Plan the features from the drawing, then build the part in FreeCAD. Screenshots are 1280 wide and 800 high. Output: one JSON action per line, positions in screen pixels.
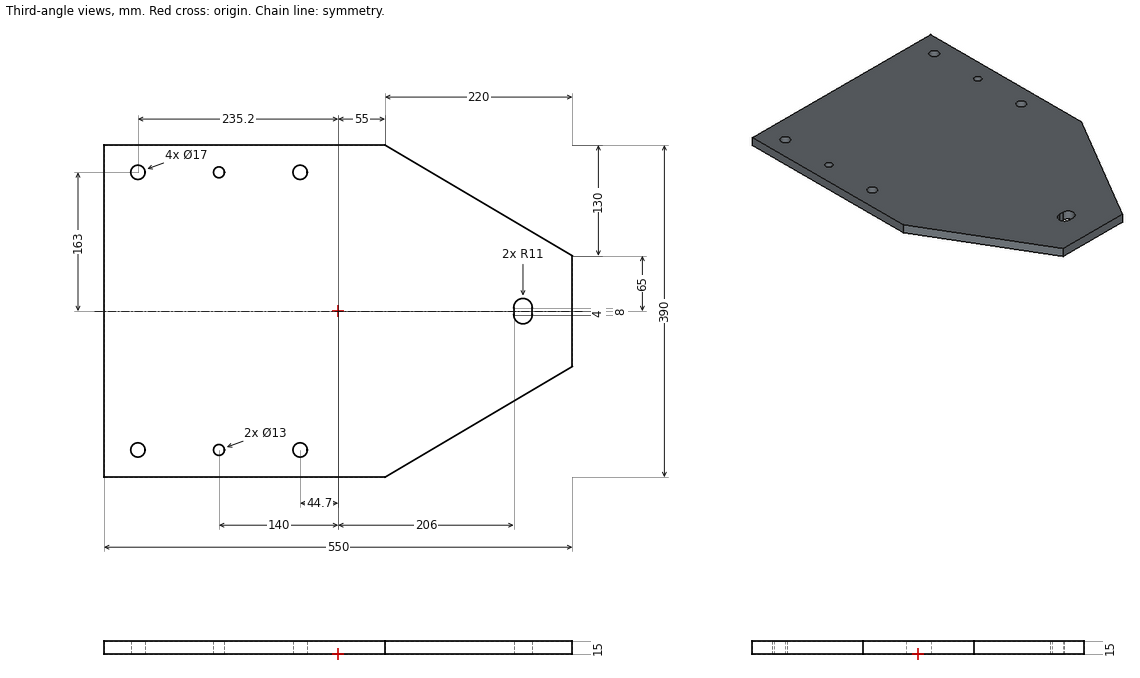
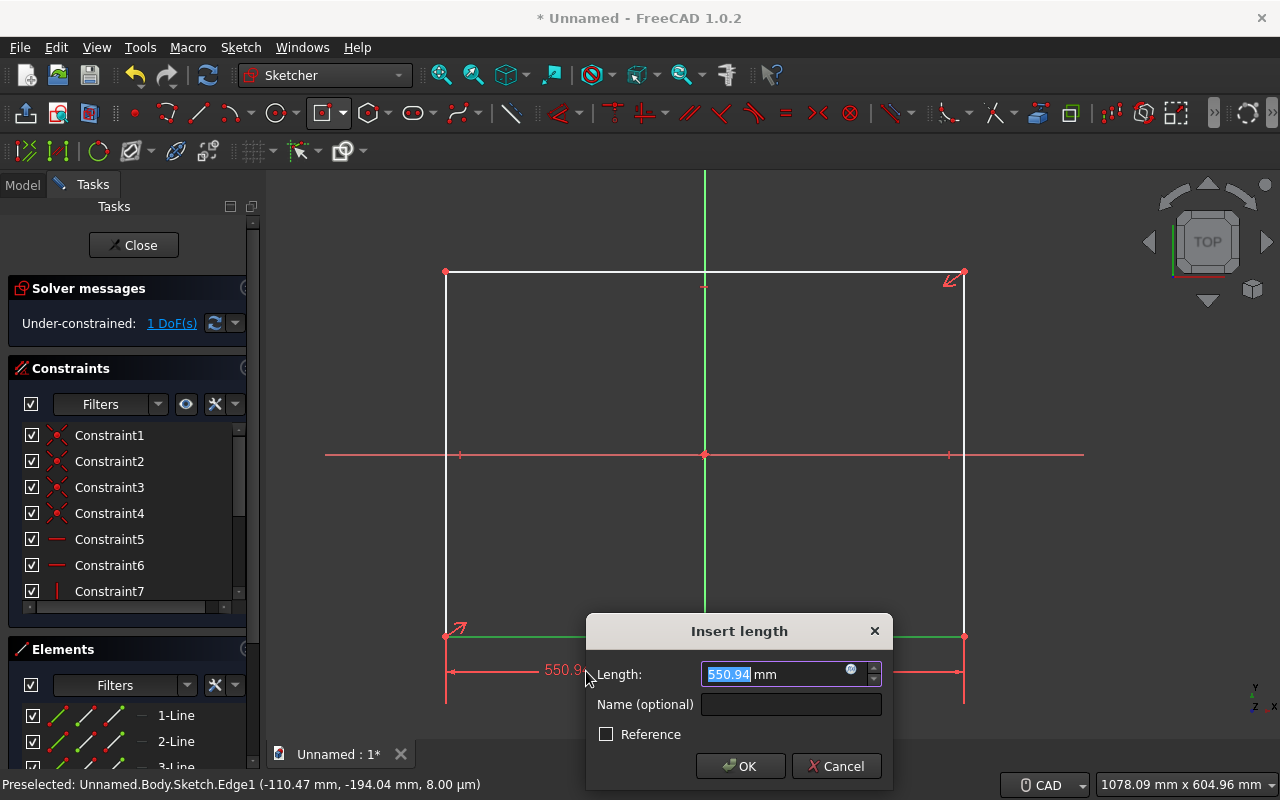
{"action": "type", "text": "550"}
{"action": "key", "text": "Return"}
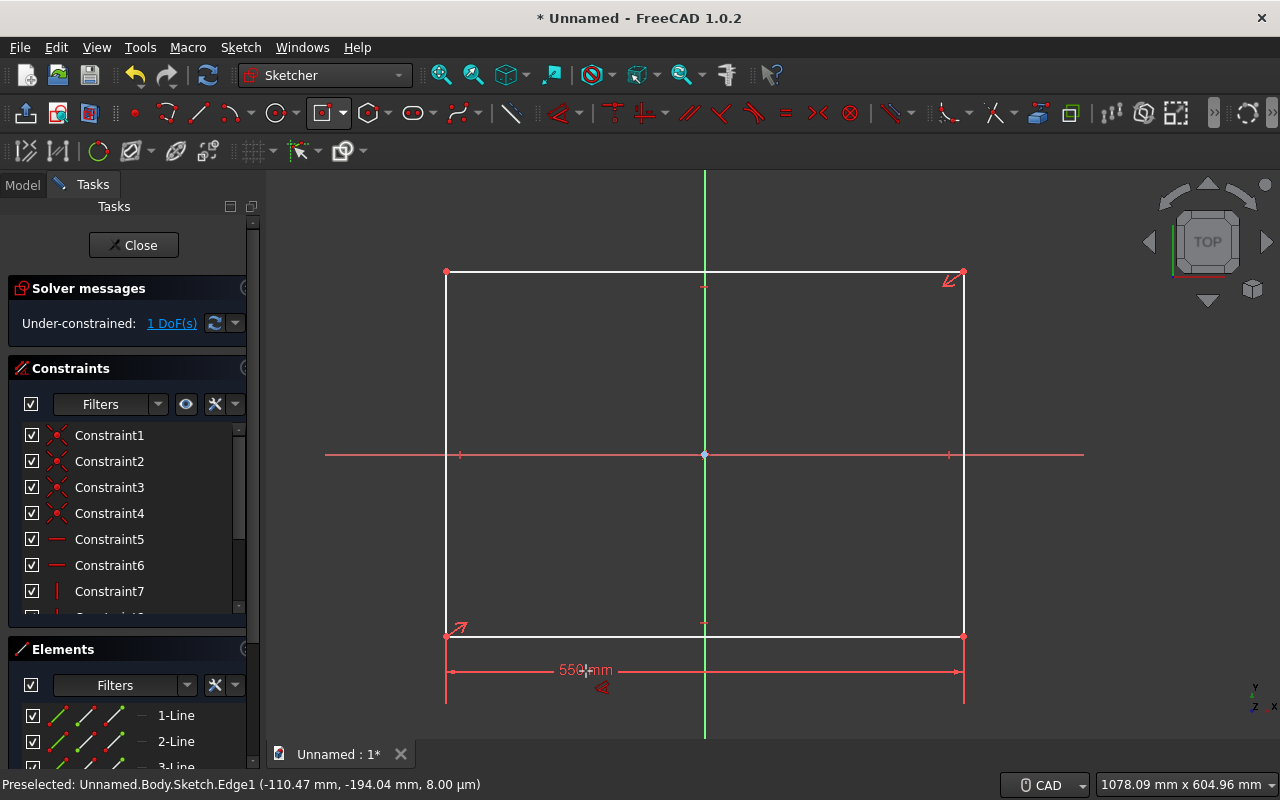
{"action": "left_click", "coordinate": [964, 527]}
{"action": "left_click", "coordinate": [998, 371]}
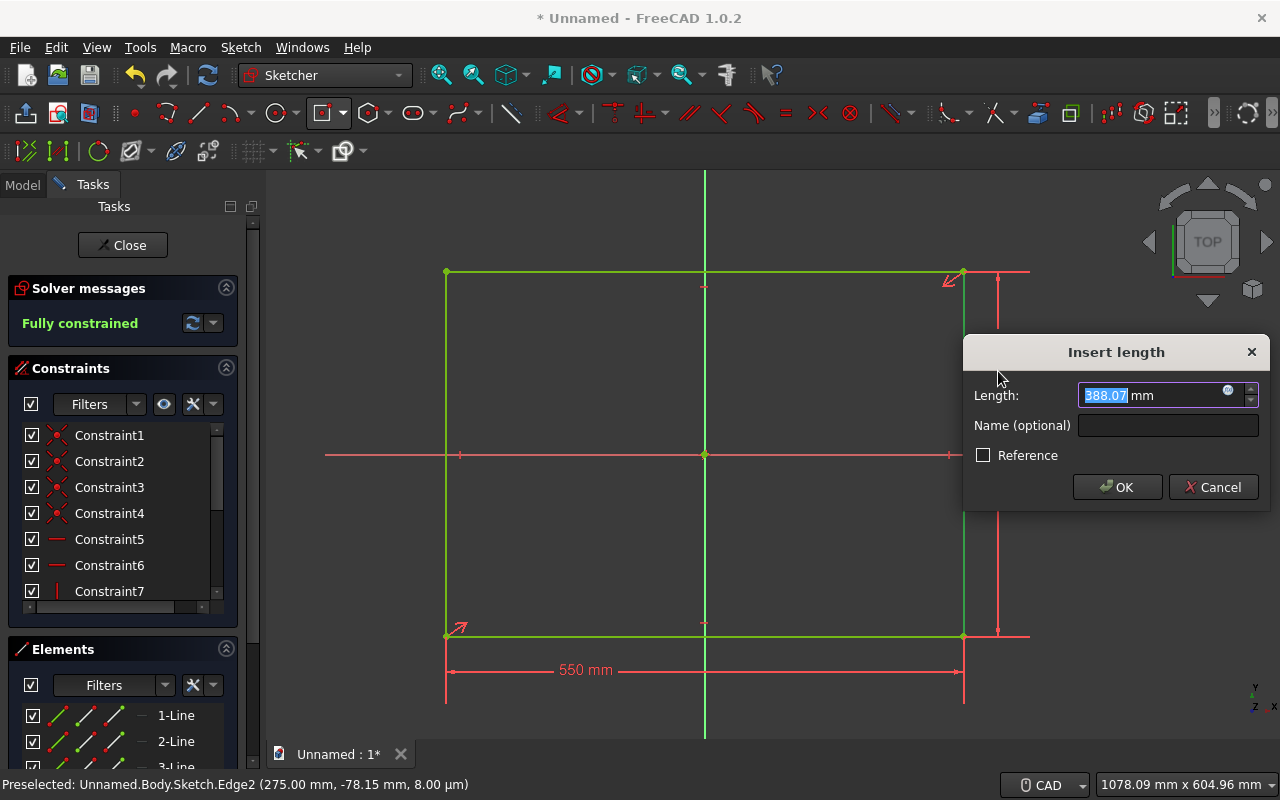
{"action": "type", "text": "390"}
{"action": "key", "text": "Return"}
{"action": "key", "text": "Escape"}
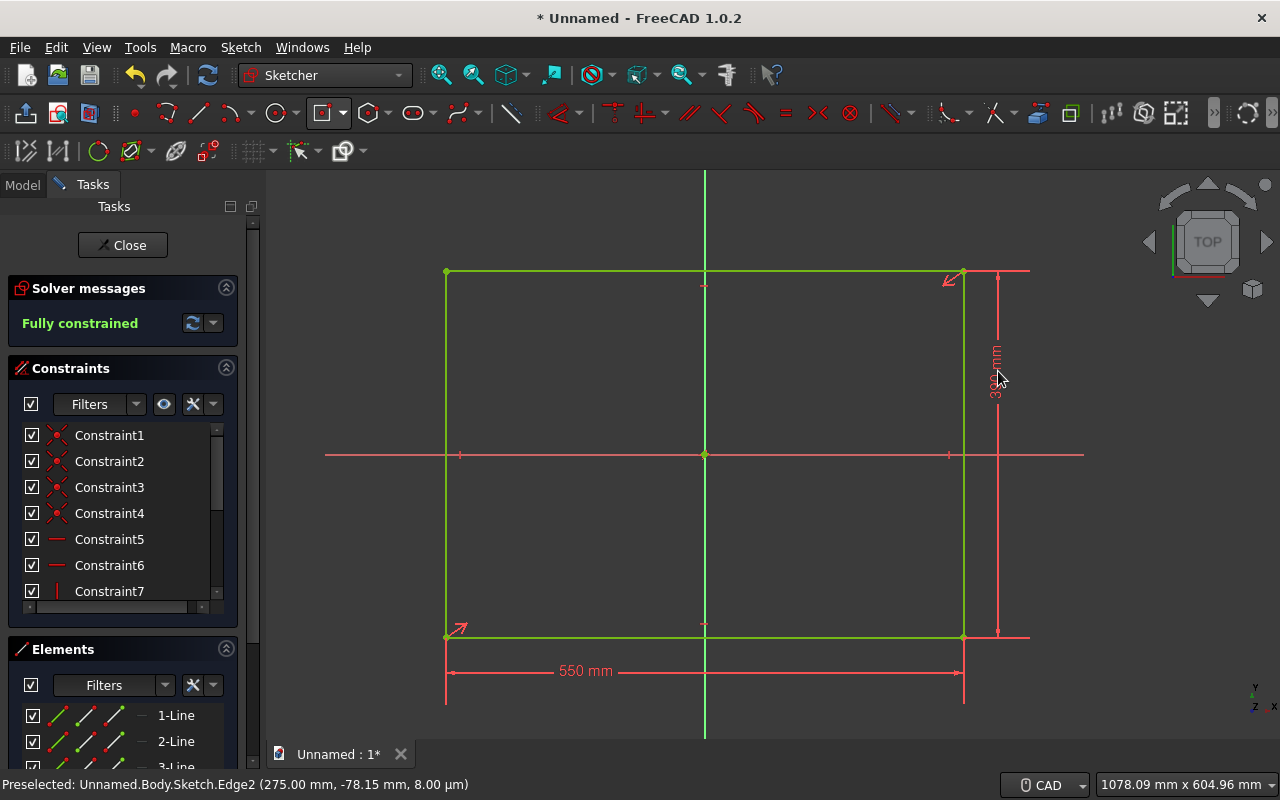
{"action": "left_click", "coordinate": [123, 245]}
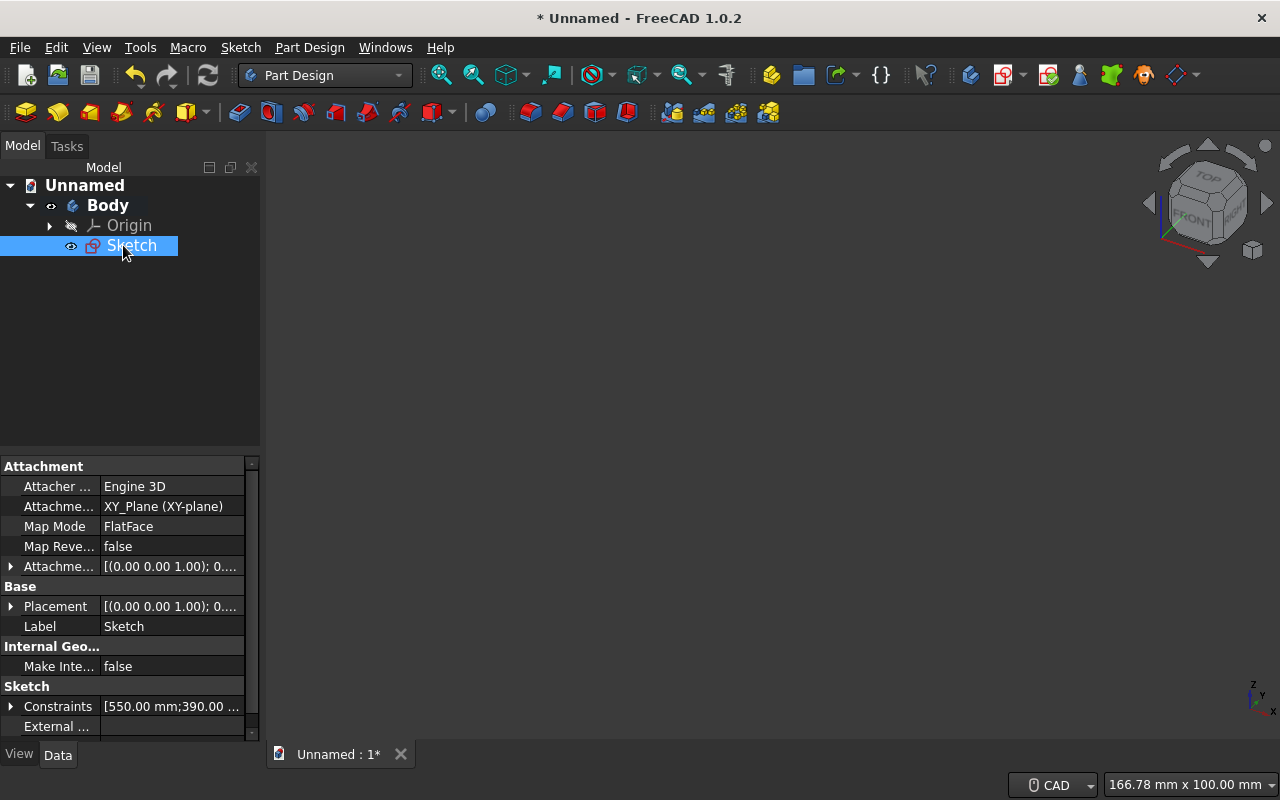
{"action": "left_click", "coordinate": [26, 112]}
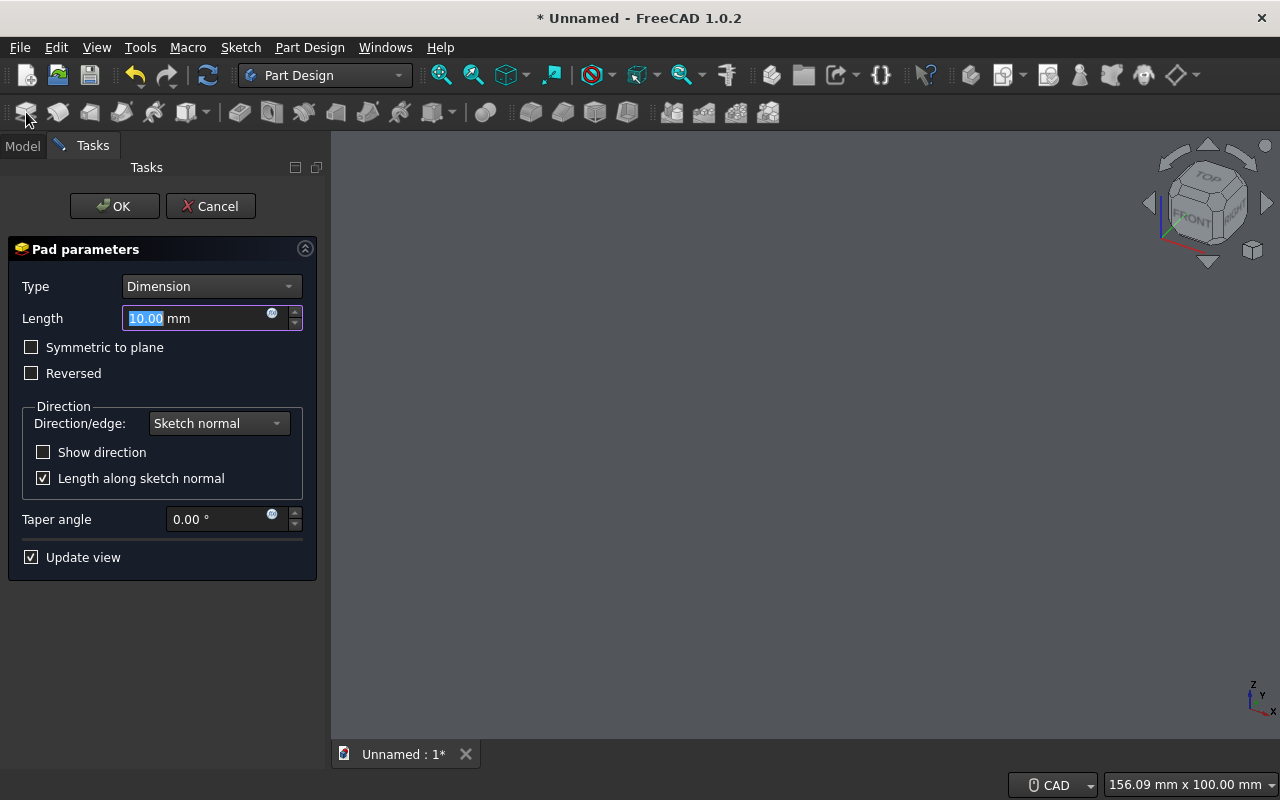
{"action": "type", "text": "15"}
{"action": "key", "text": "Tab"}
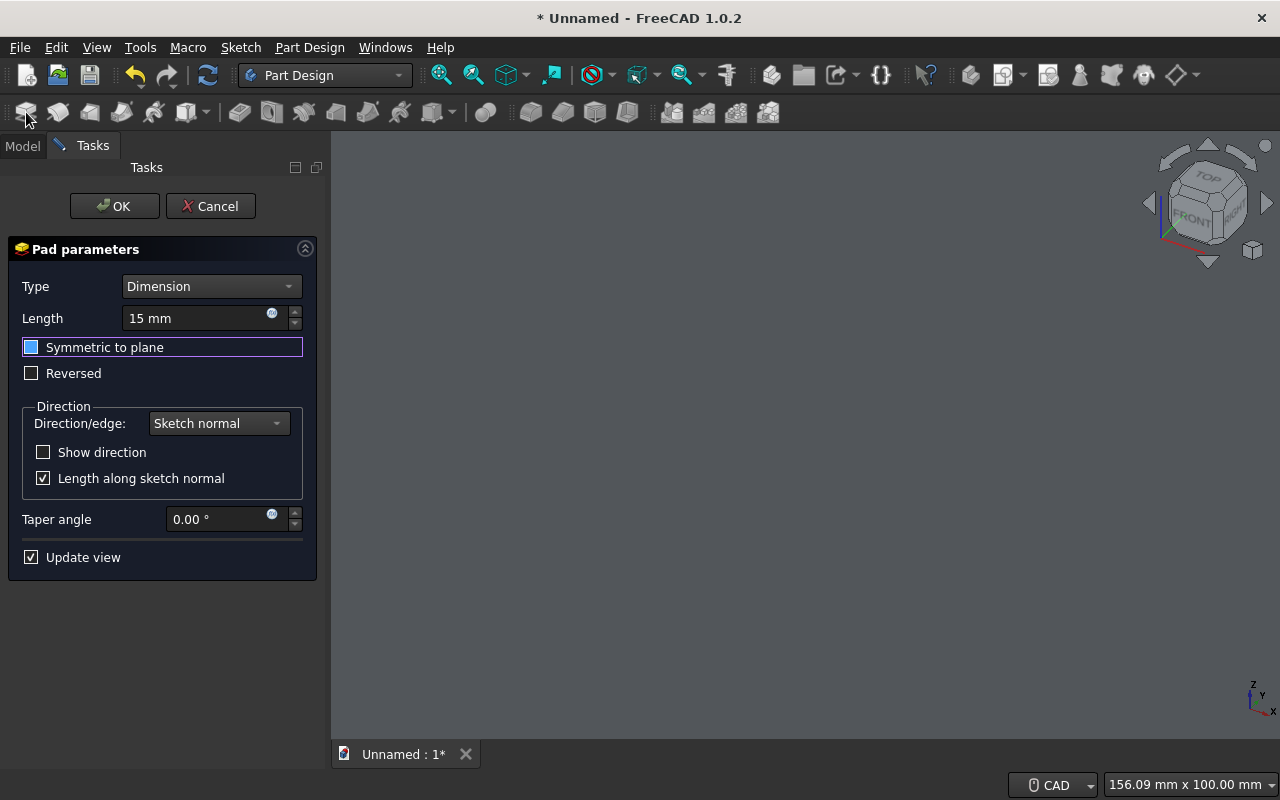
{"action": "left_click", "coordinate": [115, 206]}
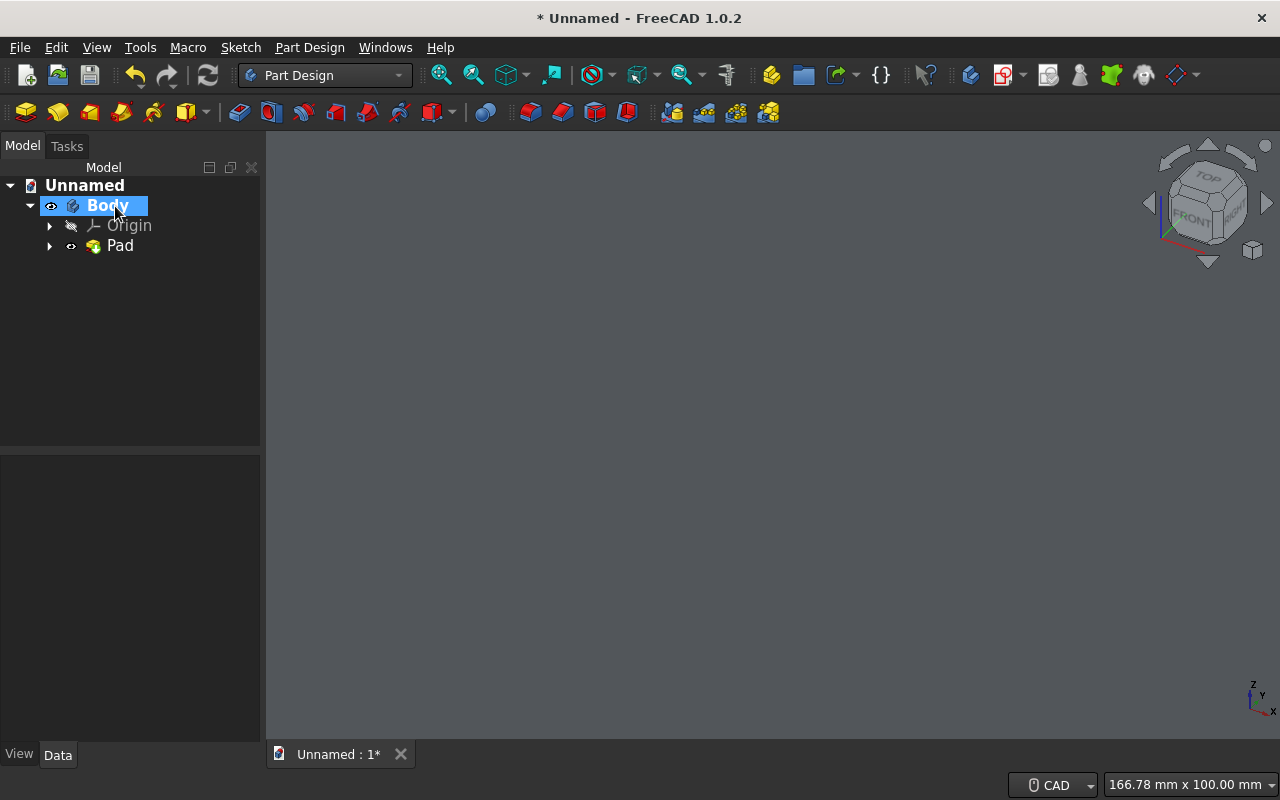
{"action": "left_click", "coordinate": [442, 76]}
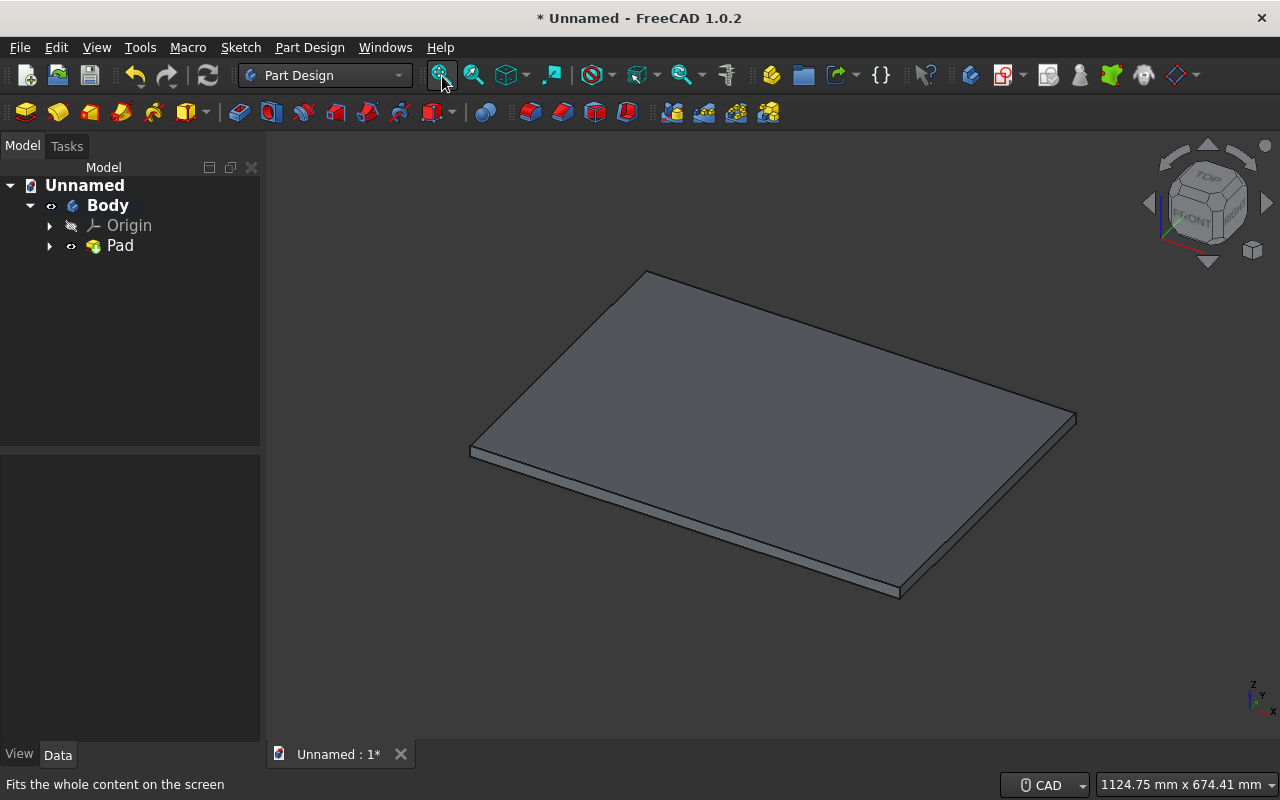
{"action": "left_click", "coordinate": [834, 449]}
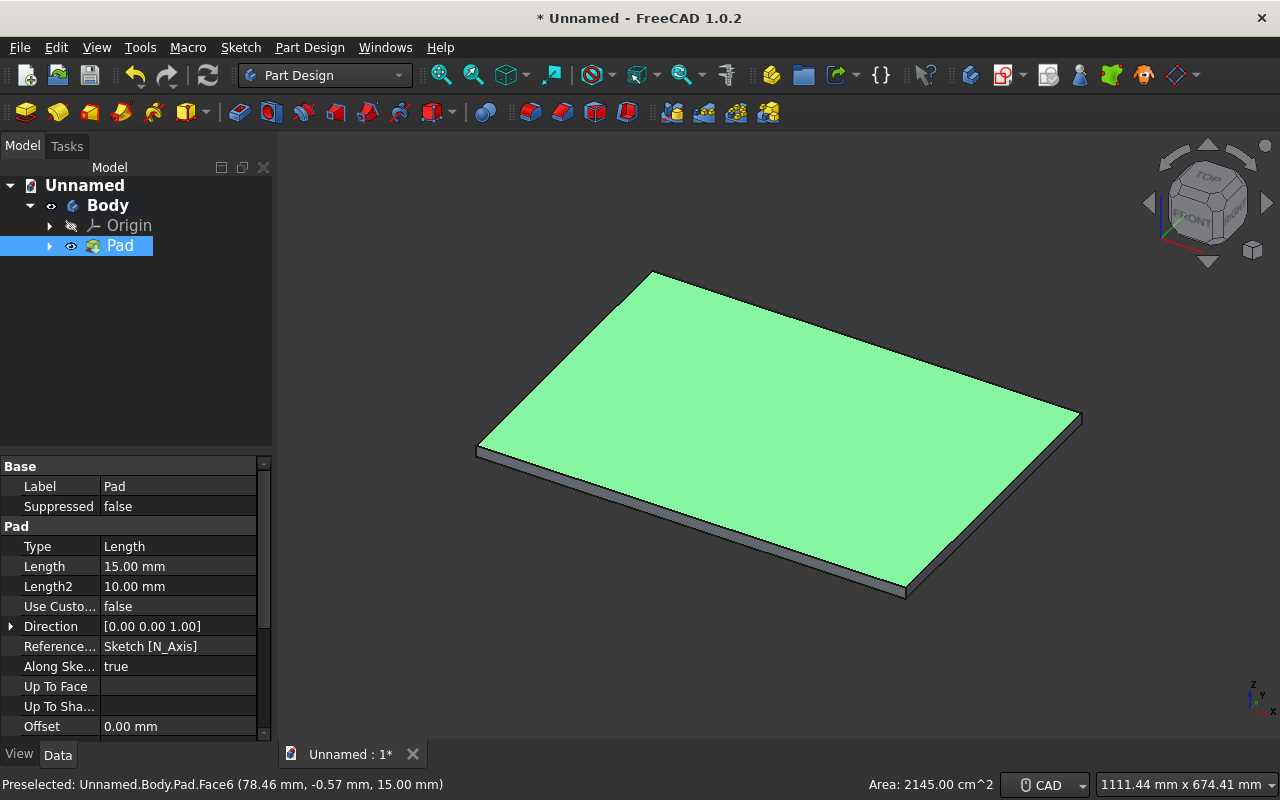
{"action": "left_click", "coordinate": [1004, 76]}